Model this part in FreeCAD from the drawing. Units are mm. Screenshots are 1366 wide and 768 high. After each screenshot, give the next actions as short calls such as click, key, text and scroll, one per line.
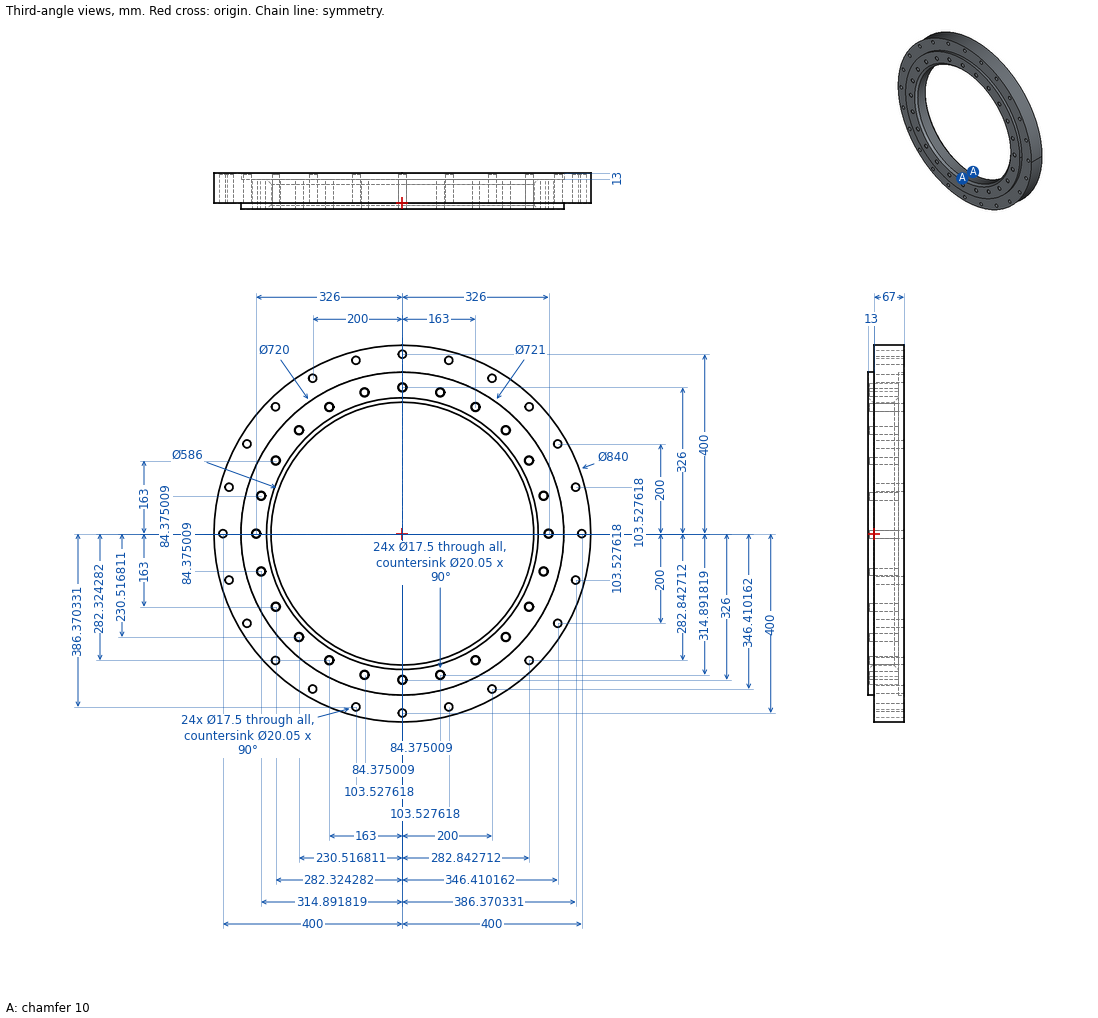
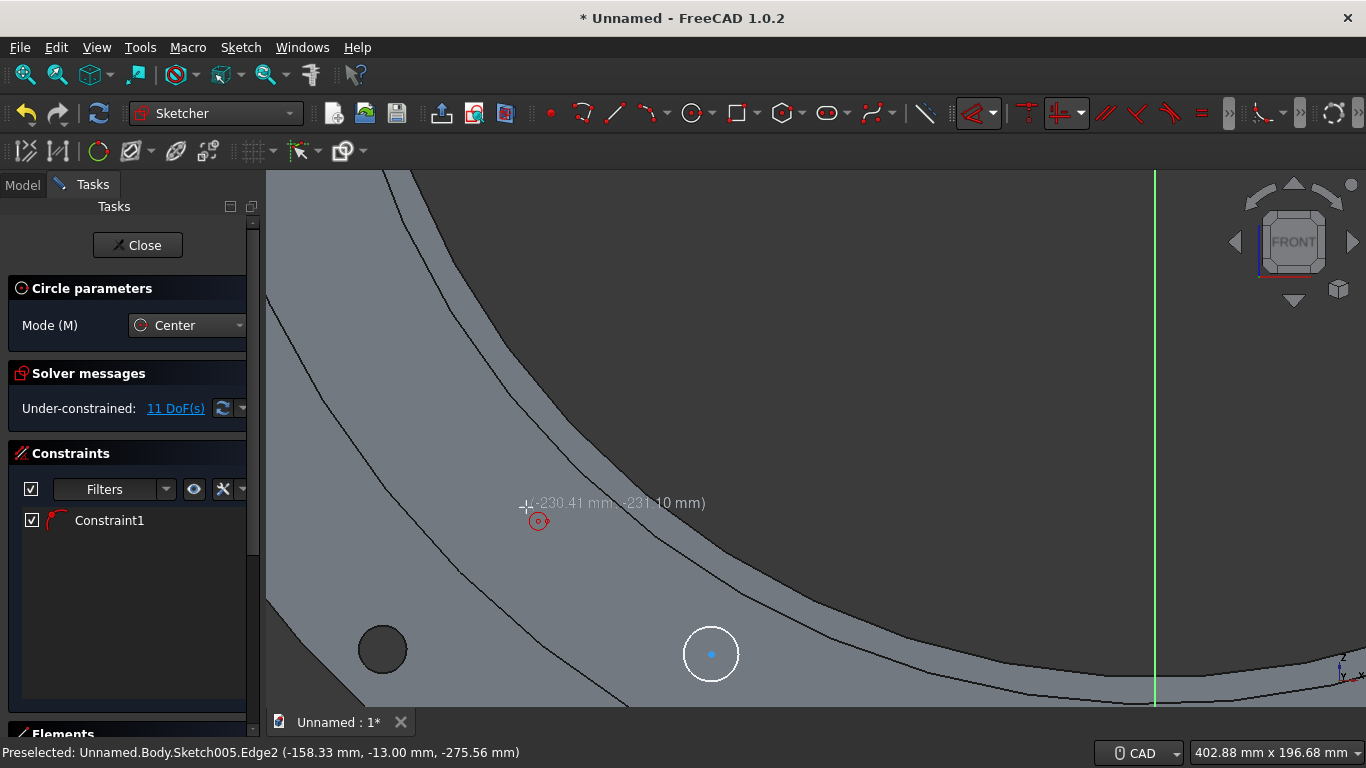
scroll(644, 580, down, 8)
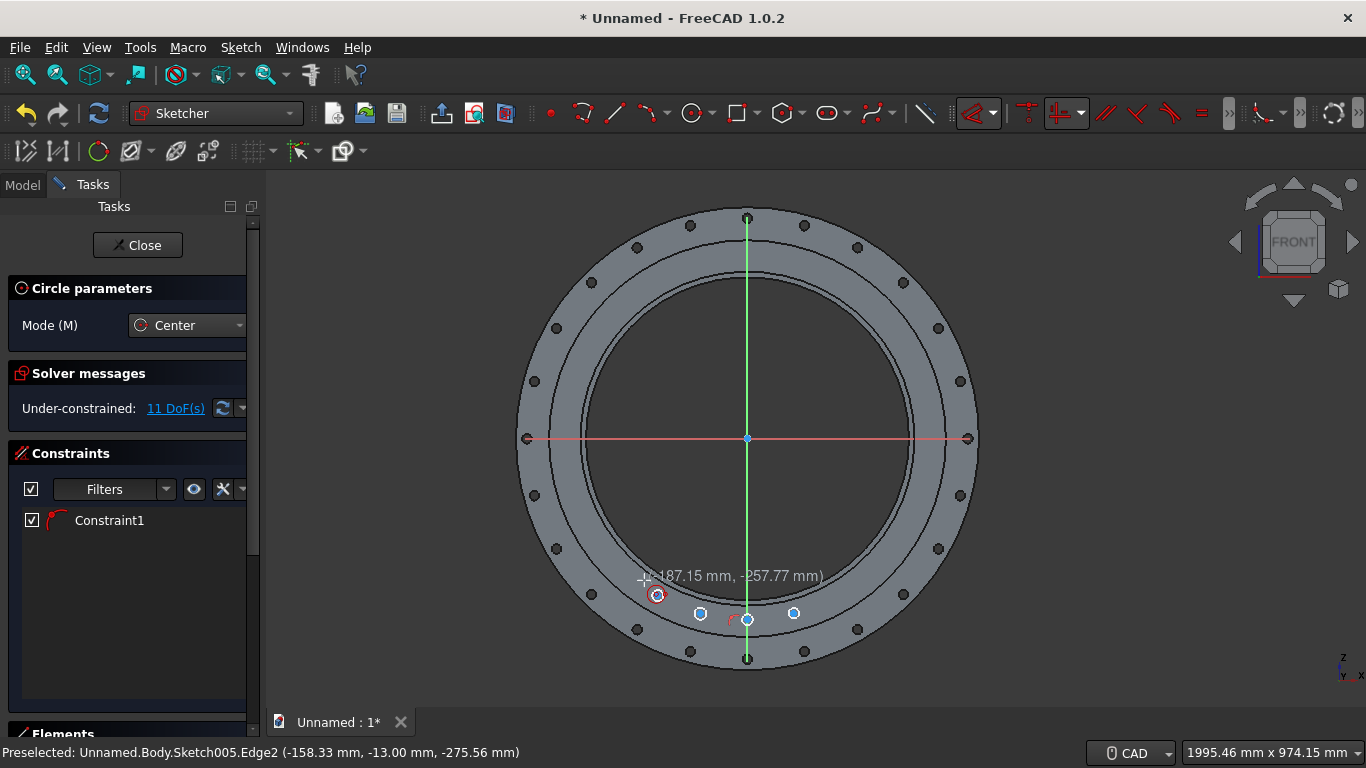
click(620, 566)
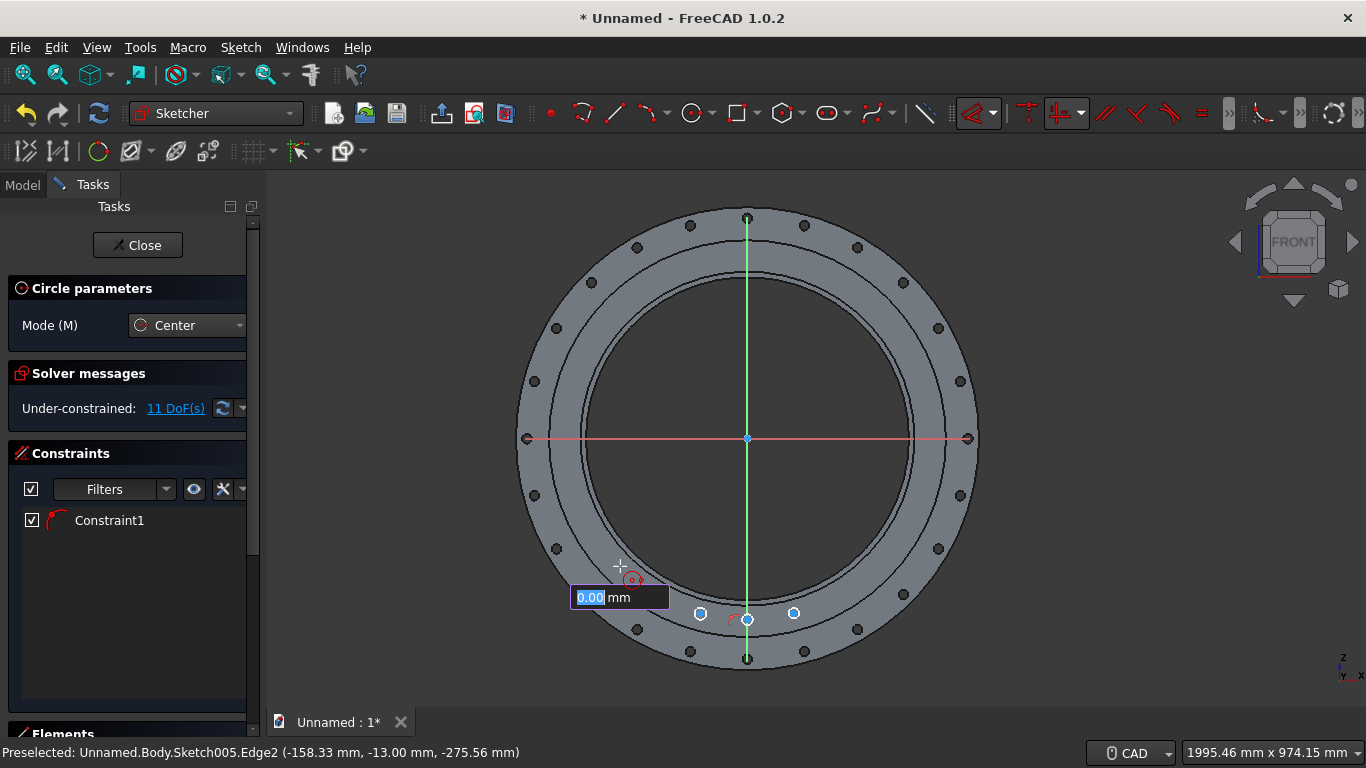
scroll(624, 562, up, 6)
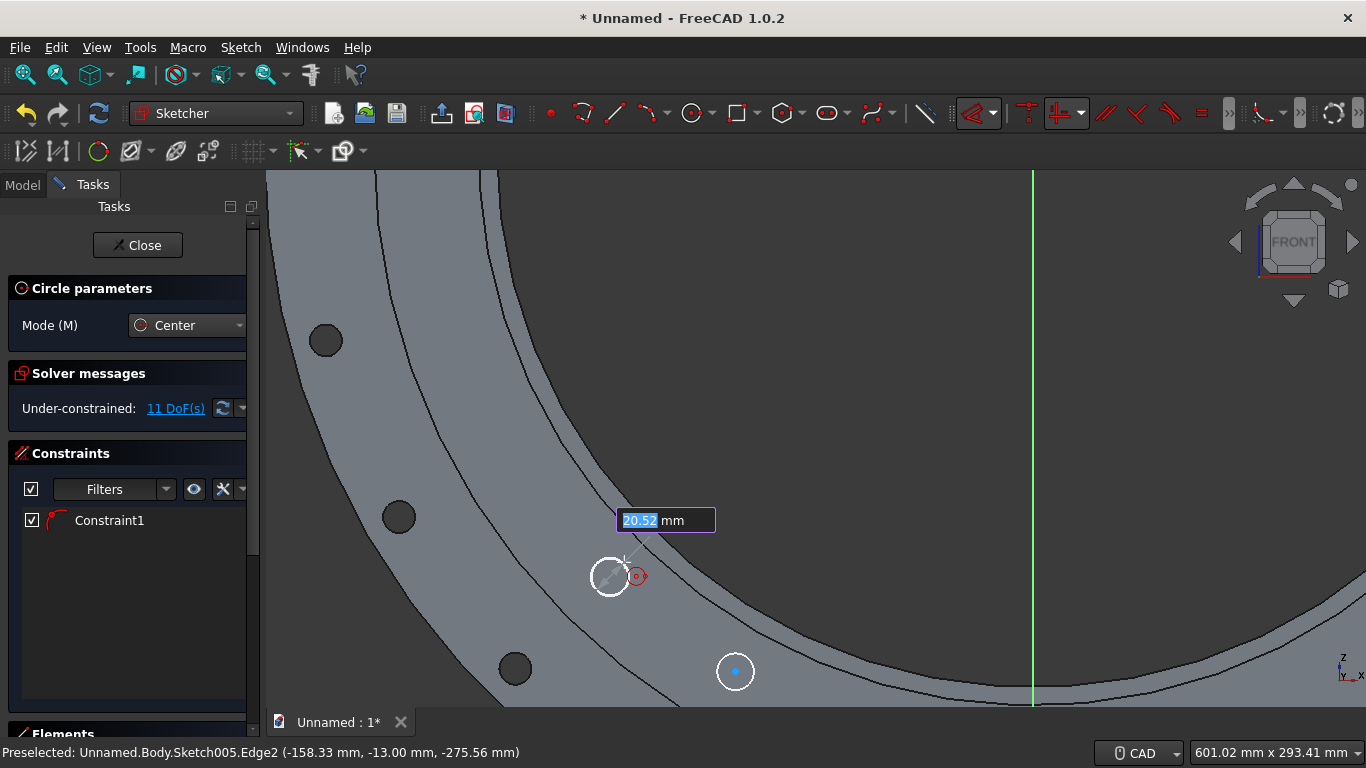
click(623, 562)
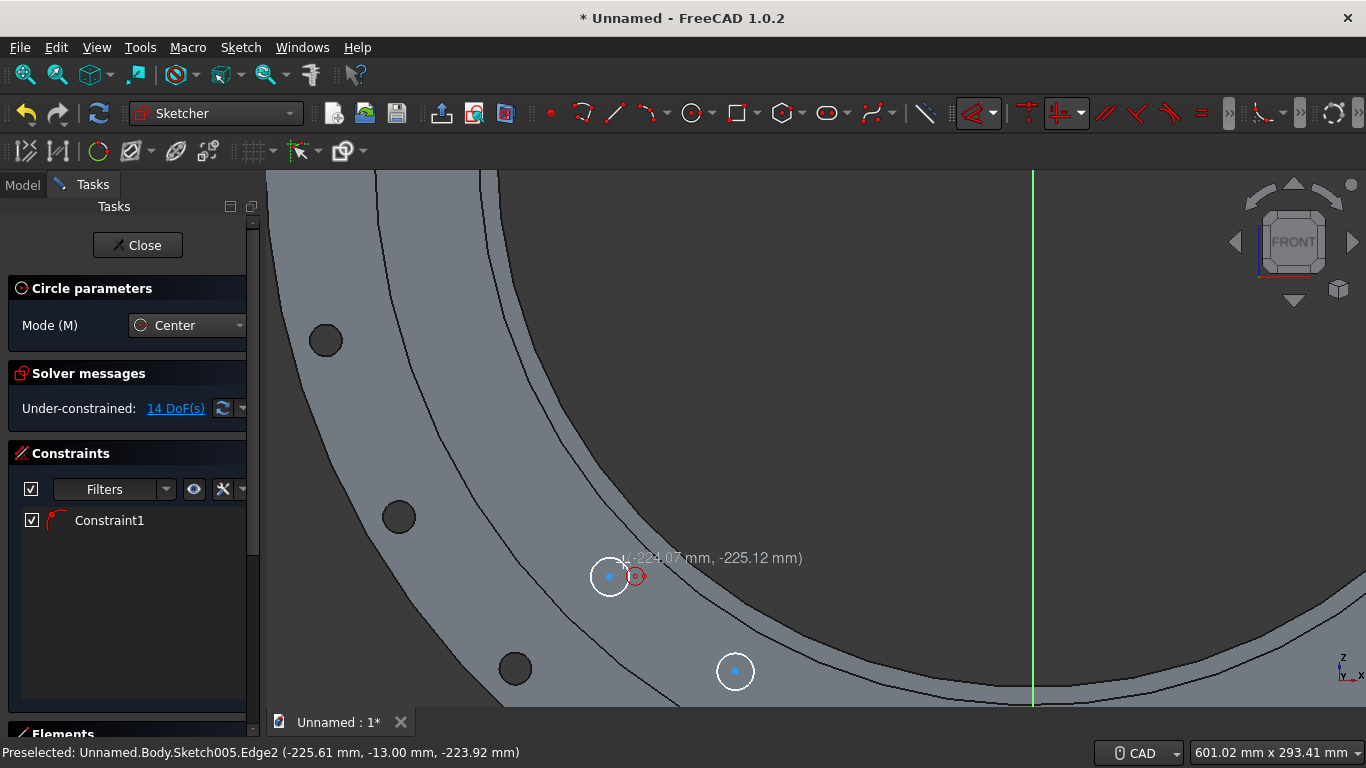
scroll(516, 449, up, 2)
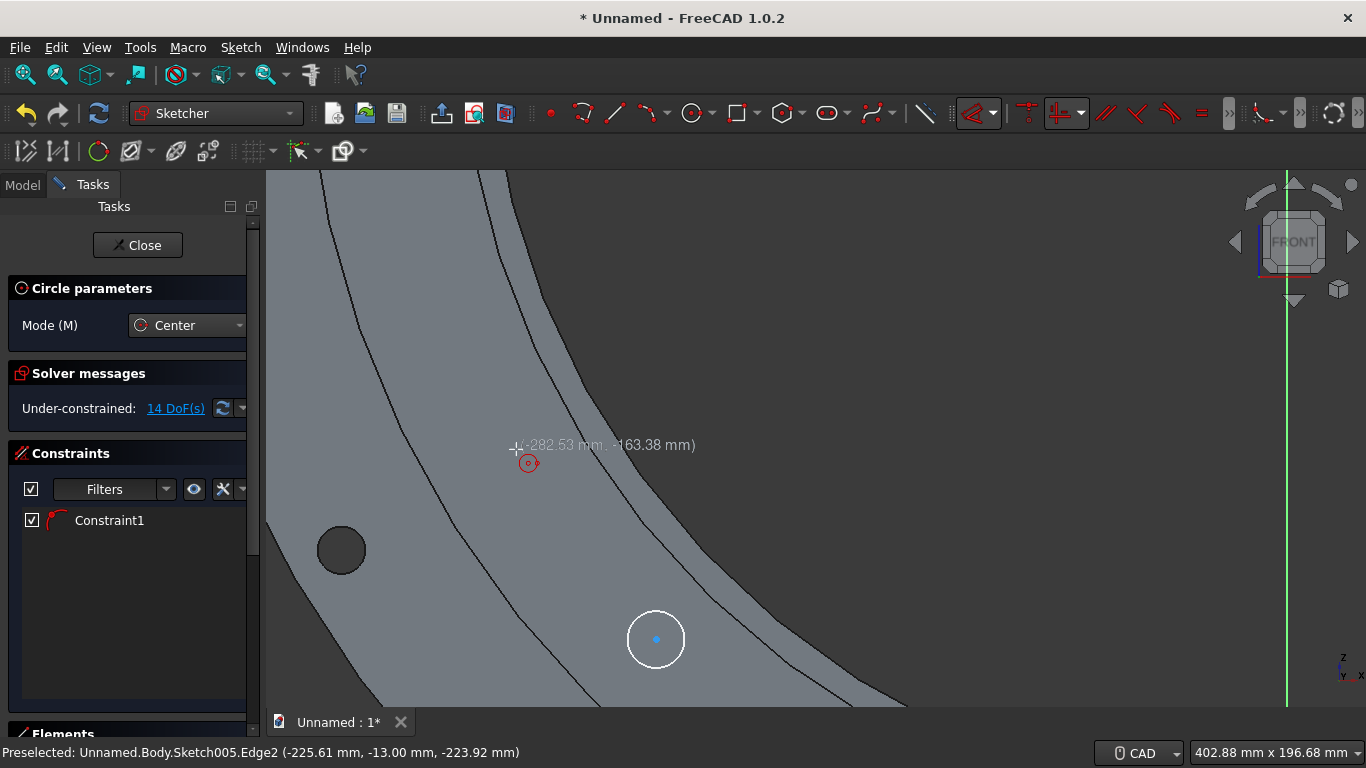
scroll(611, 548, down, 8)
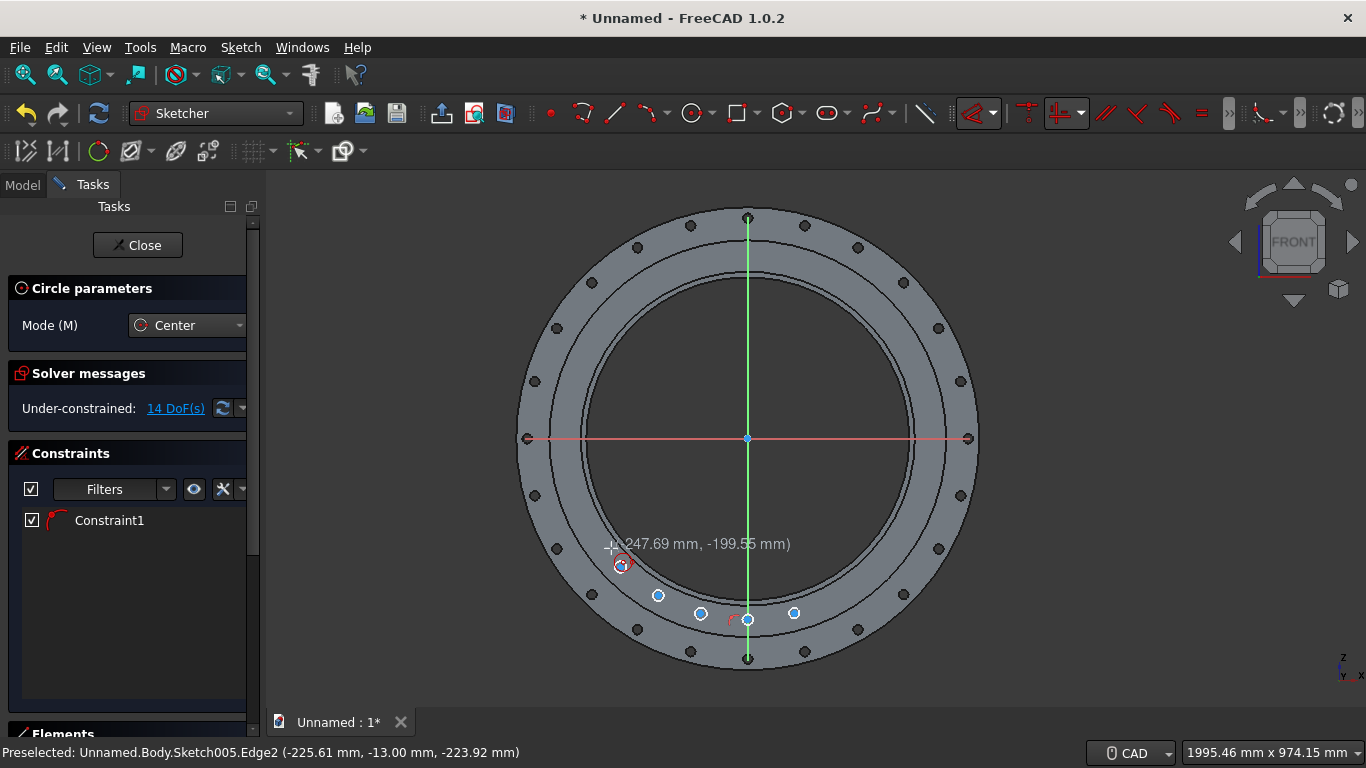
click(592, 529)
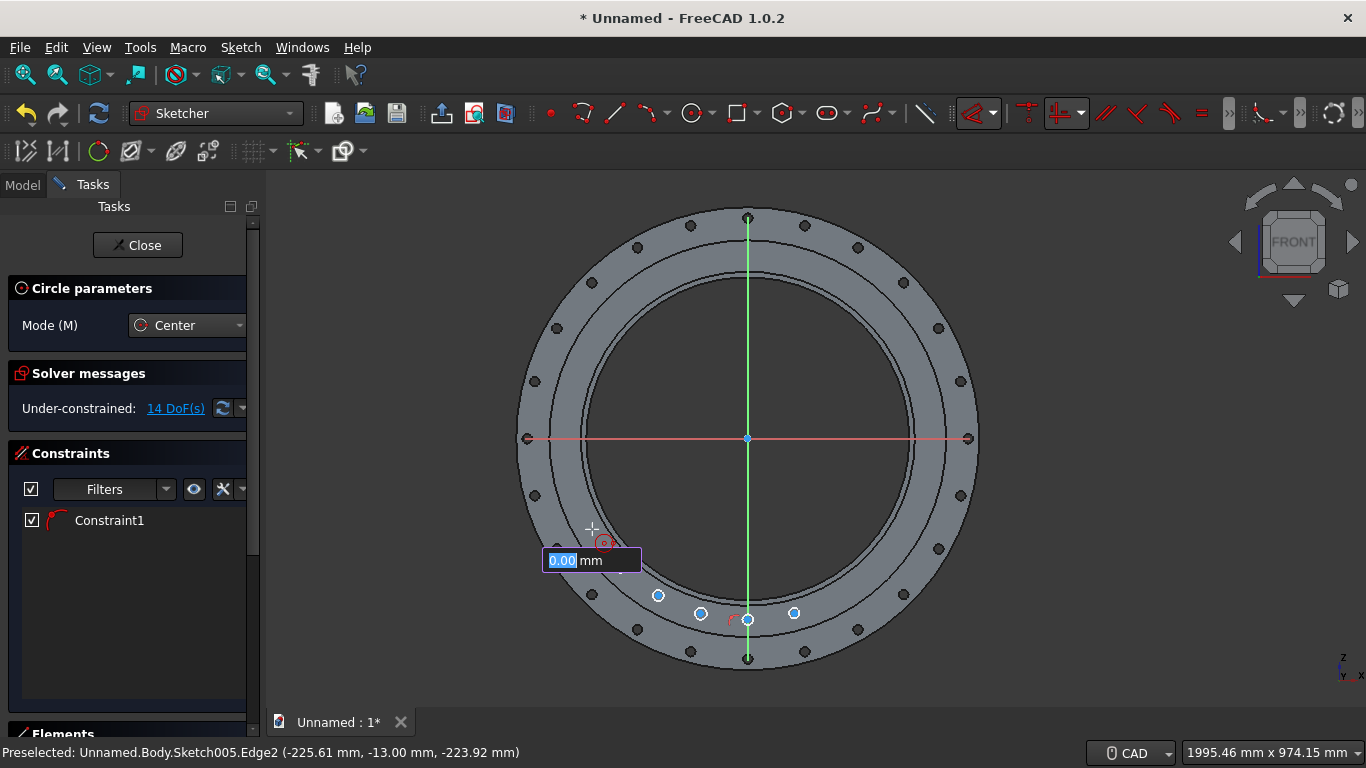
scroll(596, 525, up, 6)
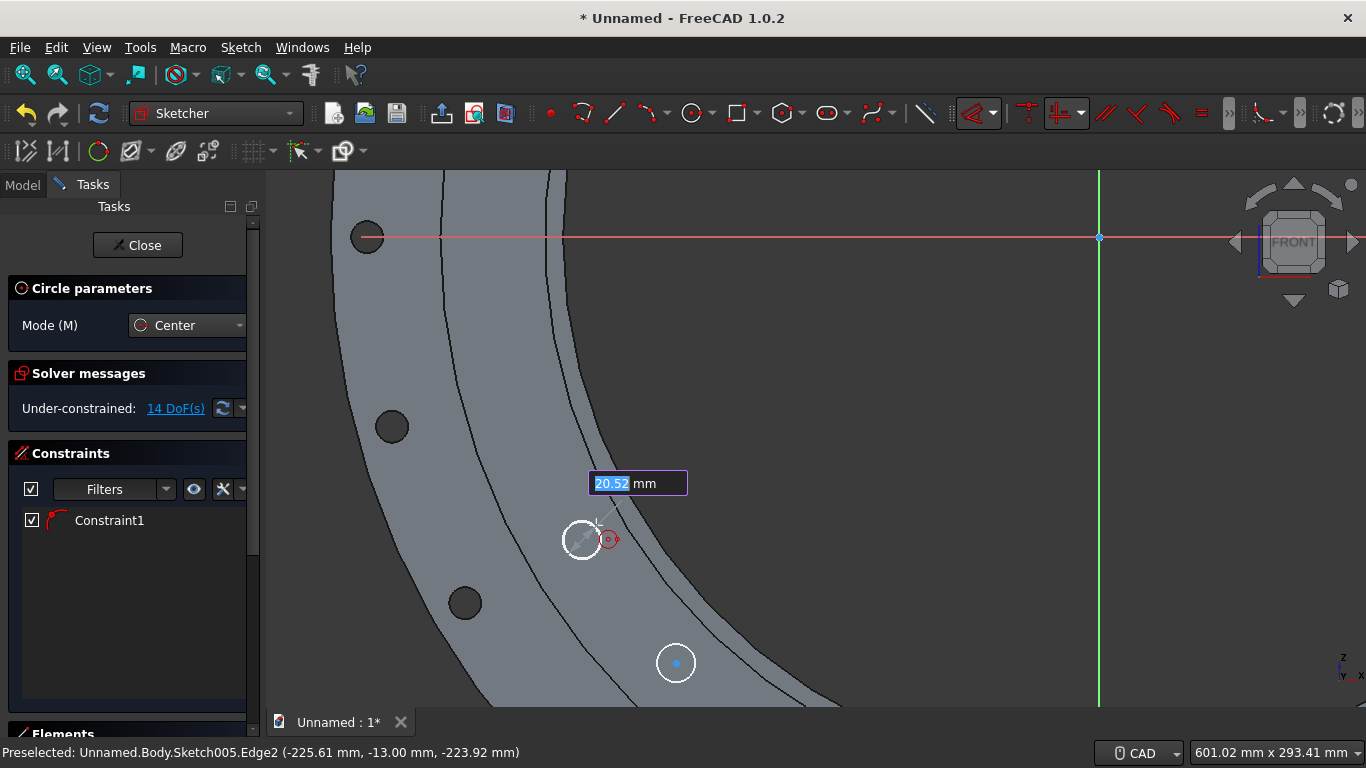
click(594, 524)